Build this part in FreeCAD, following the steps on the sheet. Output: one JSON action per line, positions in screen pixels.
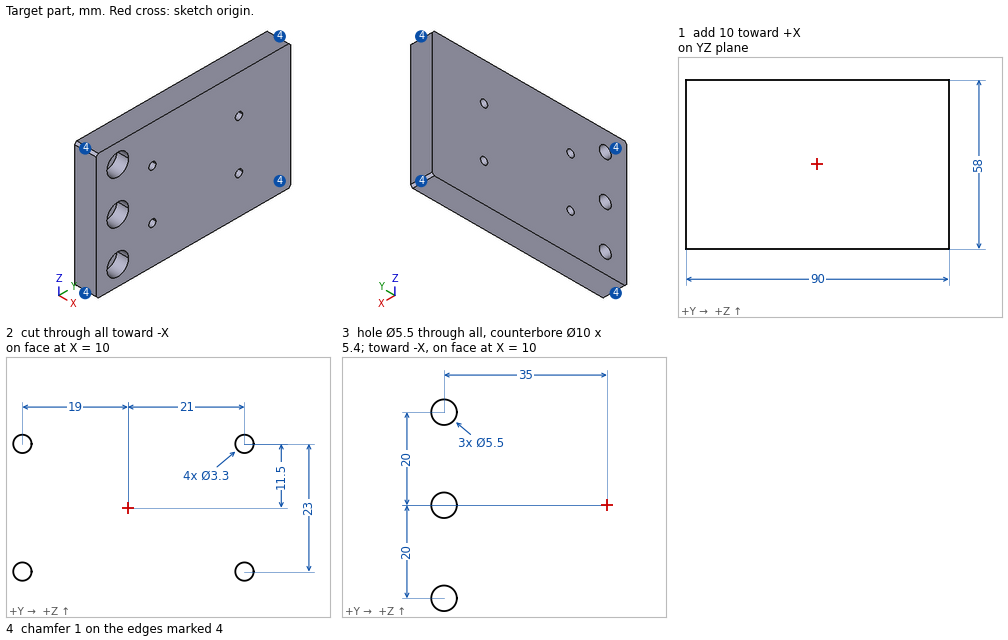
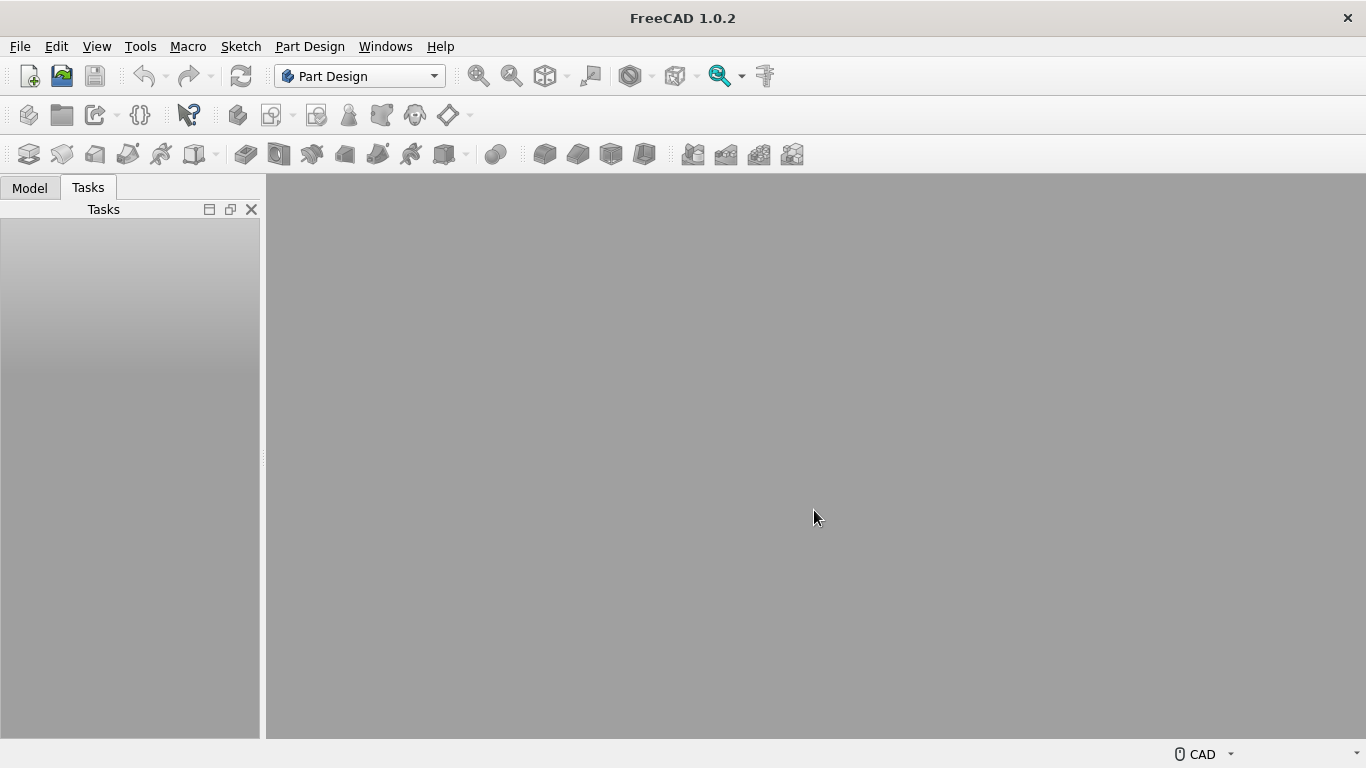
{"action": "left_click", "coordinate": [29, 76]}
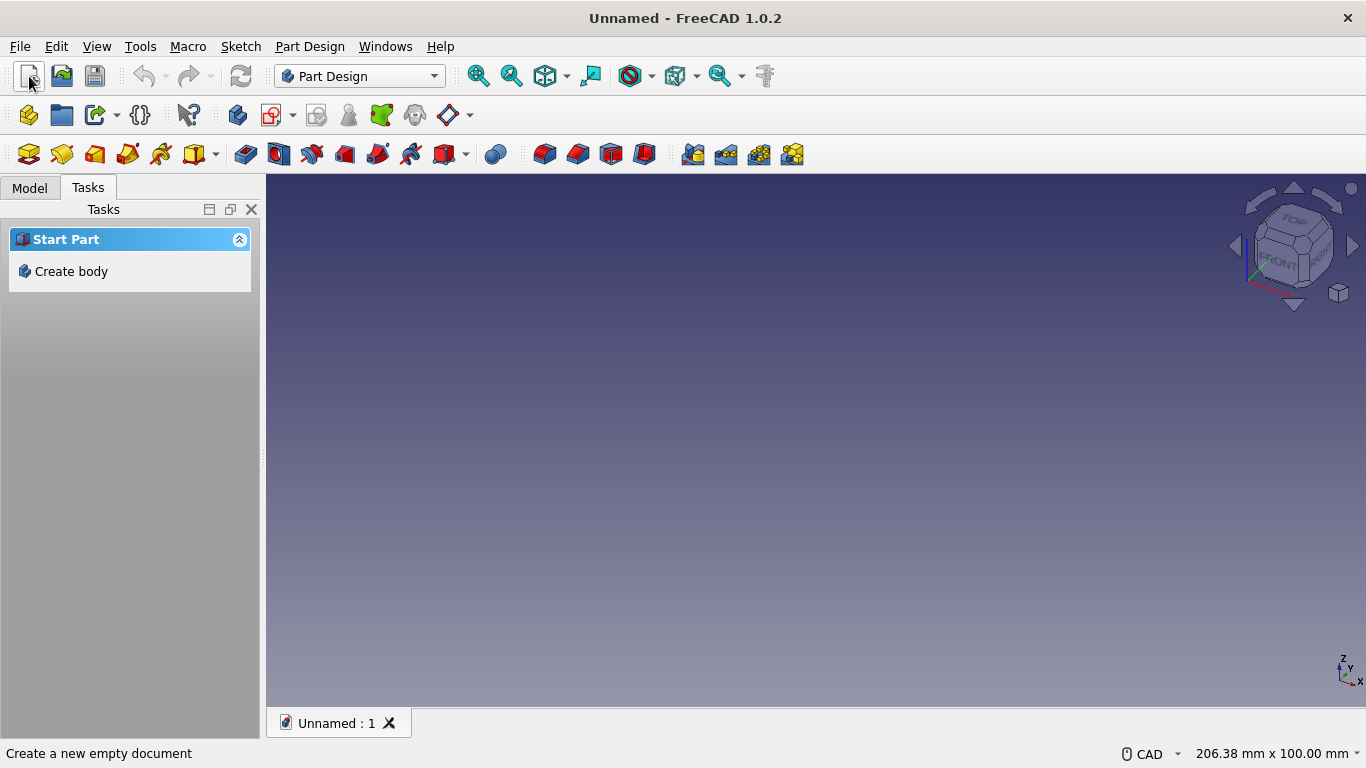
{"action": "left_click", "coordinate": [270, 116]}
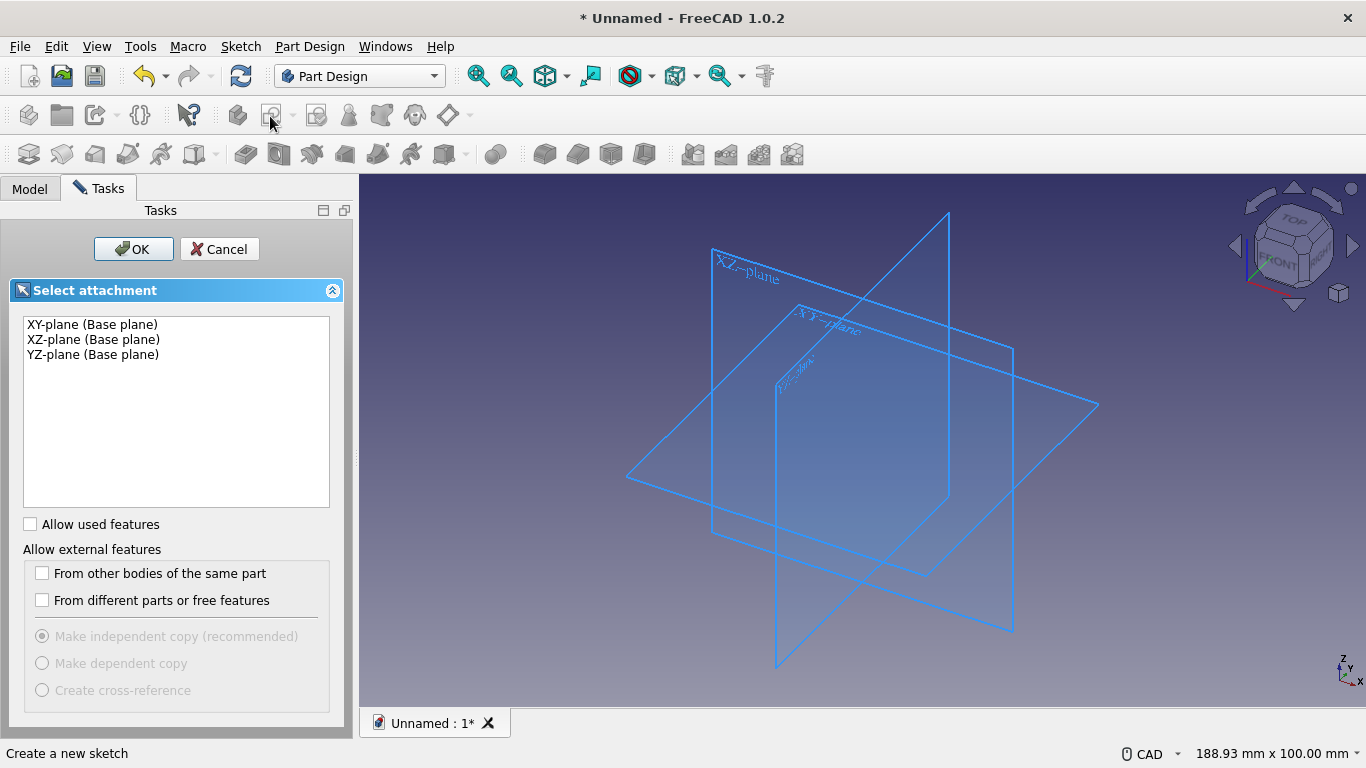
{"action": "left_click", "coordinate": [84, 354]}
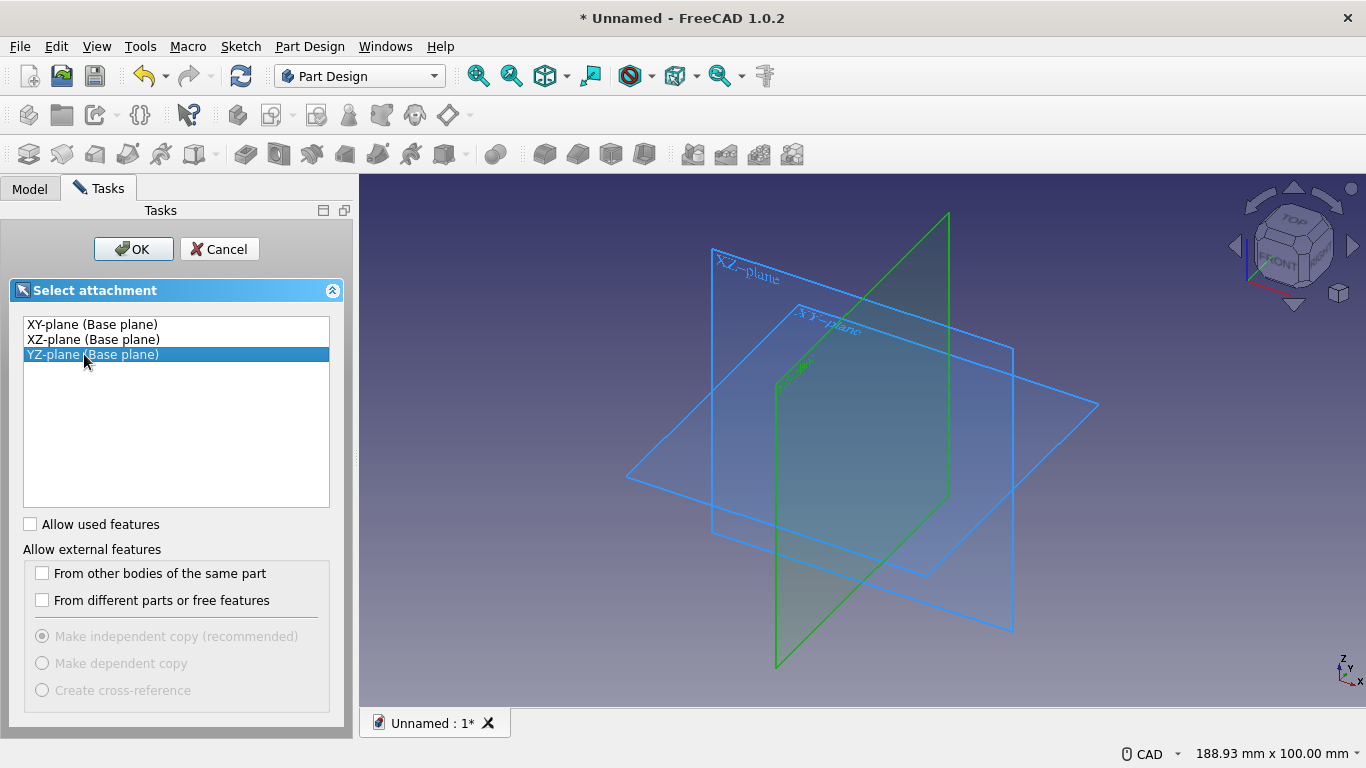
{"action": "left_click", "coordinate": [134, 249]}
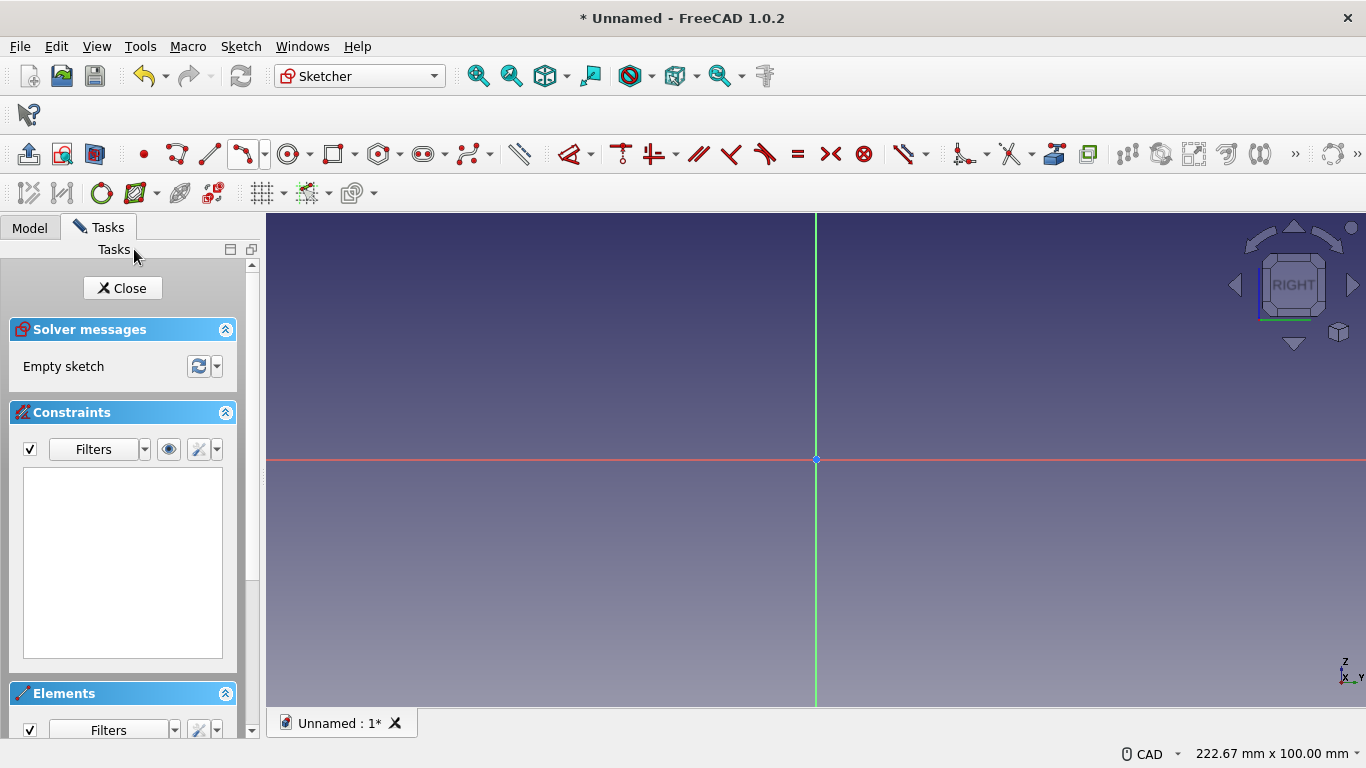
{"action": "left_click", "coordinate": [354, 154]}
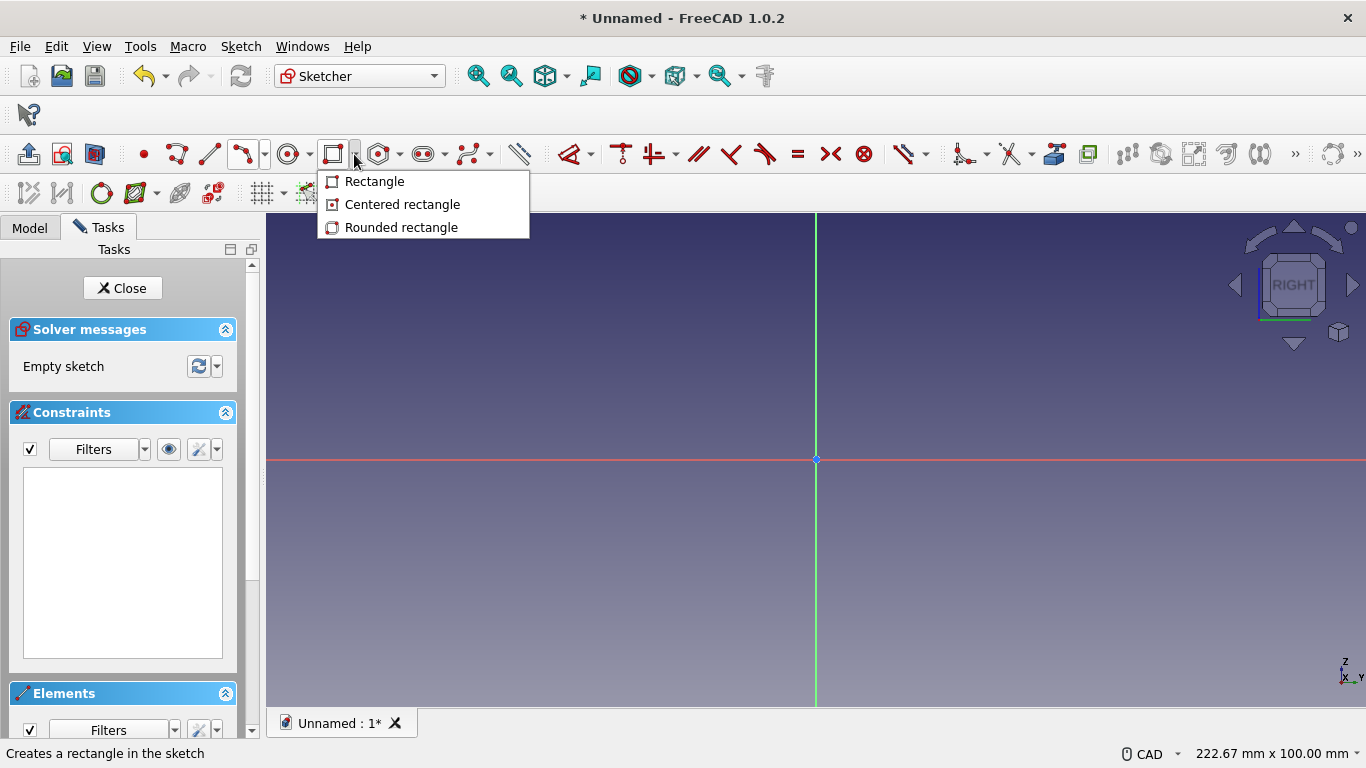
{"action": "left_click", "coordinate": [424, 204]}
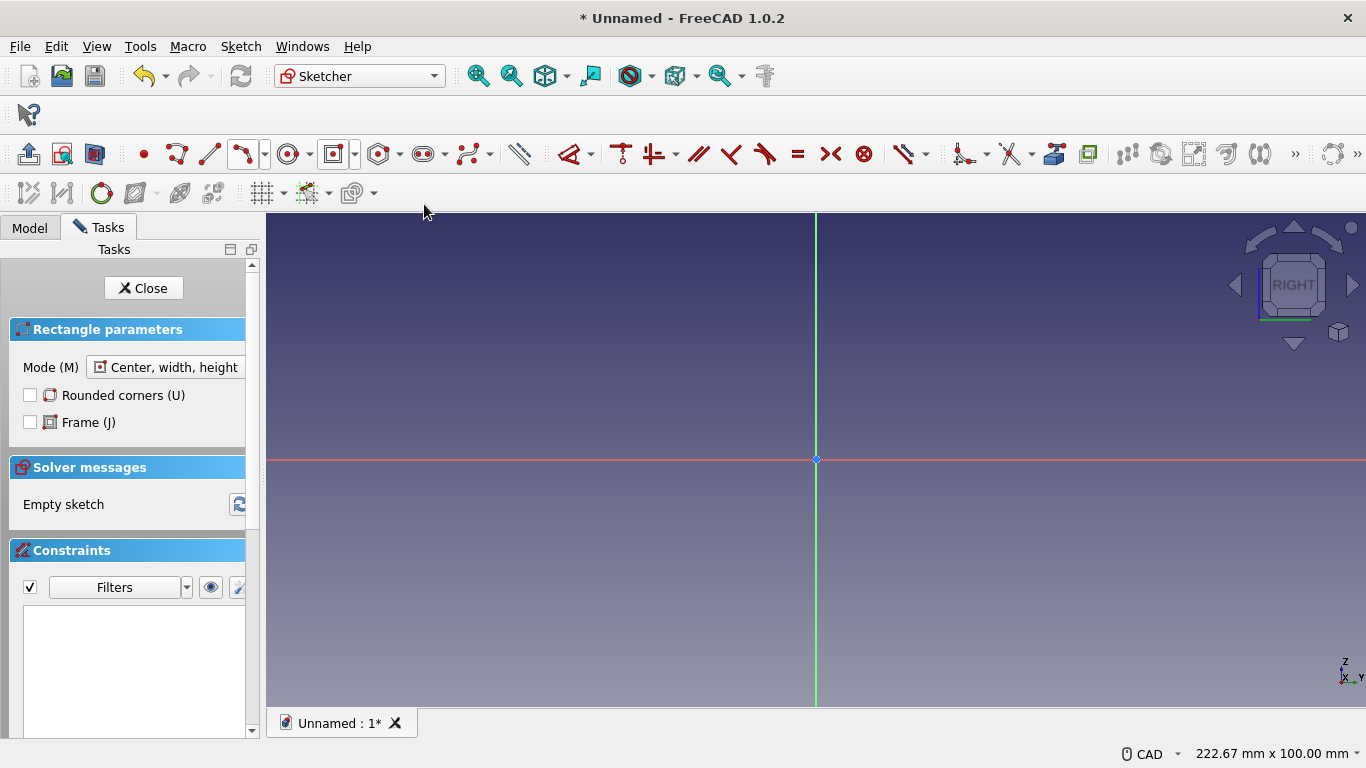
{"action": "left_click", "coordinate": [816, 460]}
{"action": "mouse_move", "coordinate": [1038, 317]}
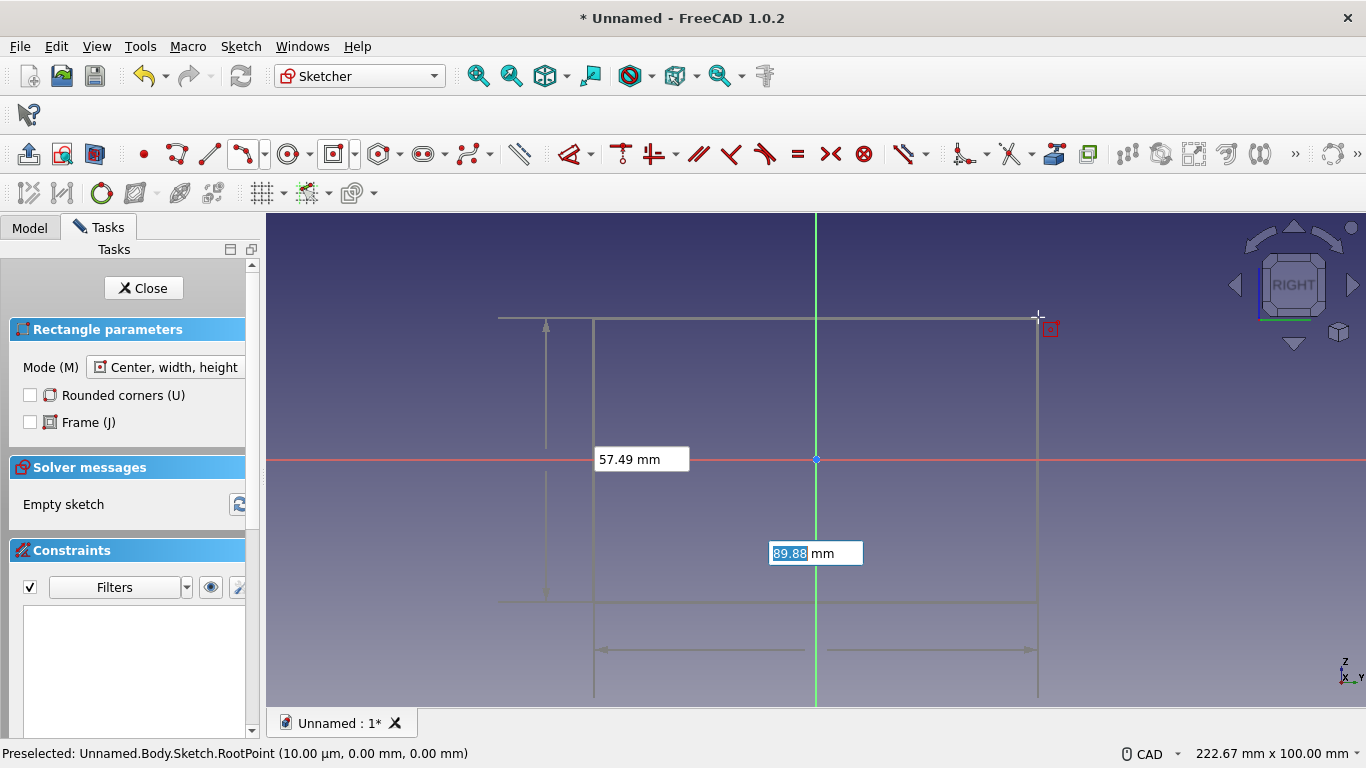
{"action": "type", "text": "90"}
{"action": "key", "text": "Tab"}
{"action": "type", "text": "58"}
{"action": "key", "text": "Return"}
{"action": "key", "text": "Escape"}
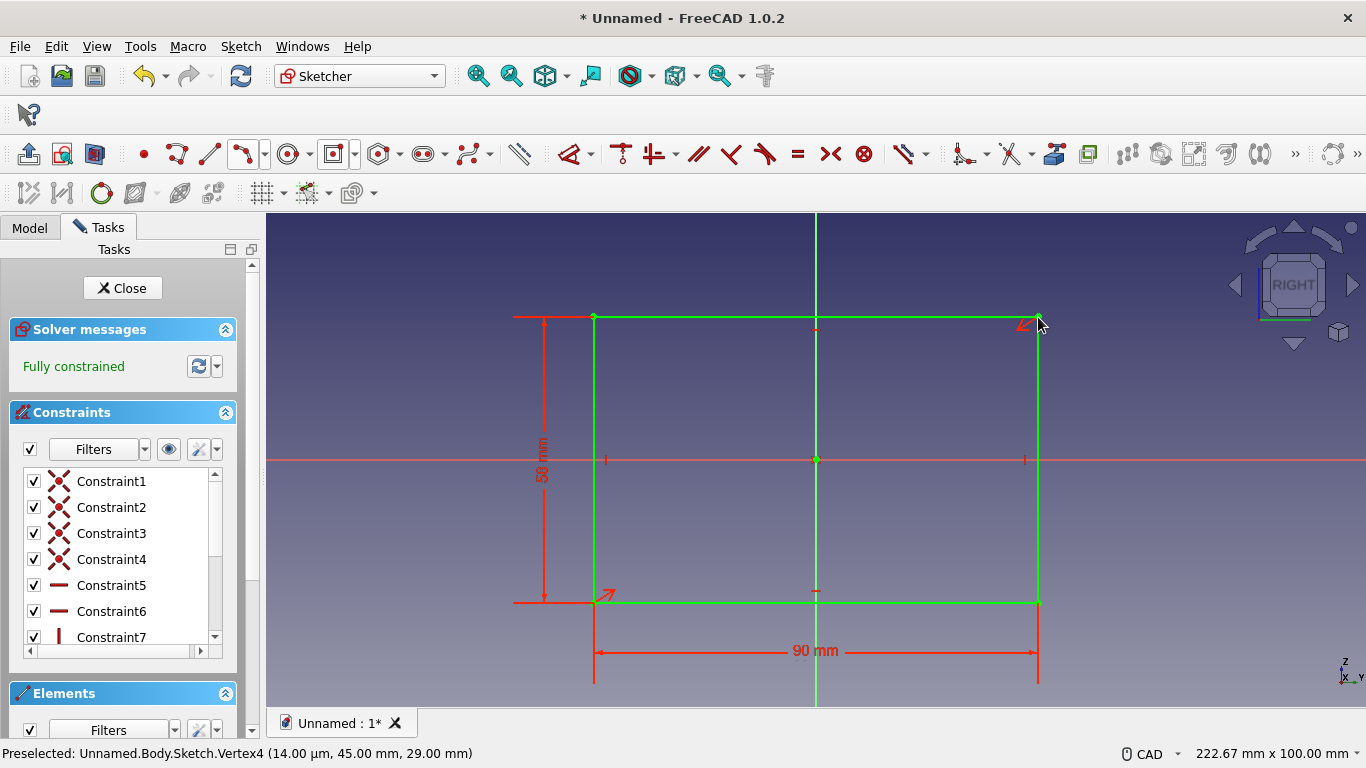
{"action": "left_click", "coordinate": [123, 288]}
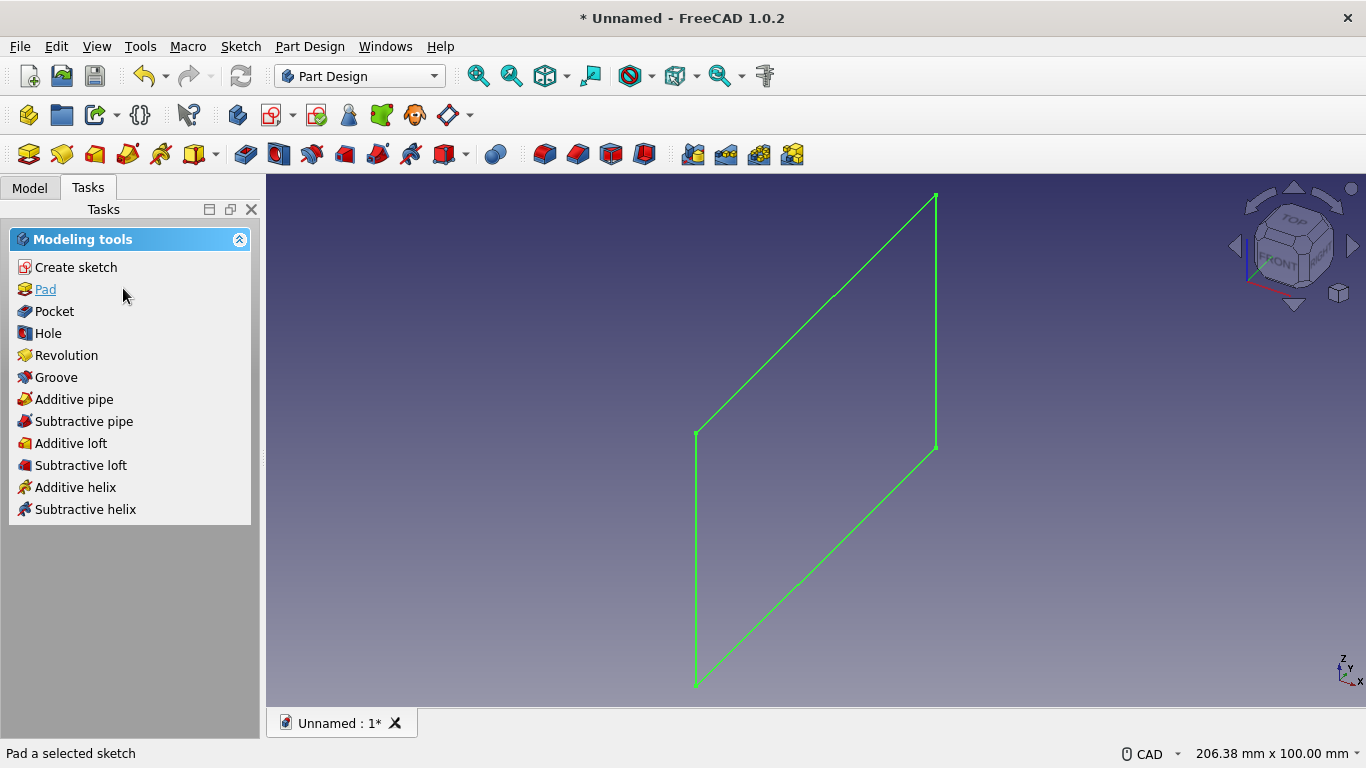
{"action": "left_click", "coordinate": [29, 154]}